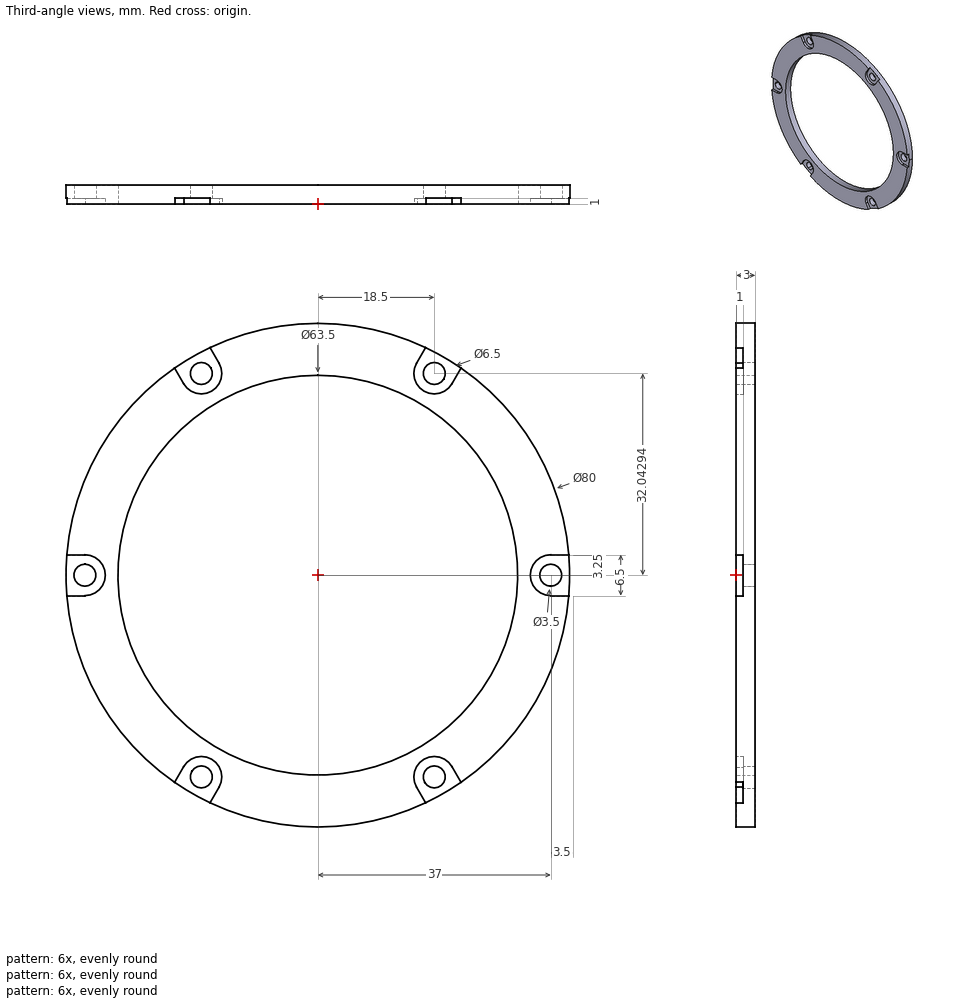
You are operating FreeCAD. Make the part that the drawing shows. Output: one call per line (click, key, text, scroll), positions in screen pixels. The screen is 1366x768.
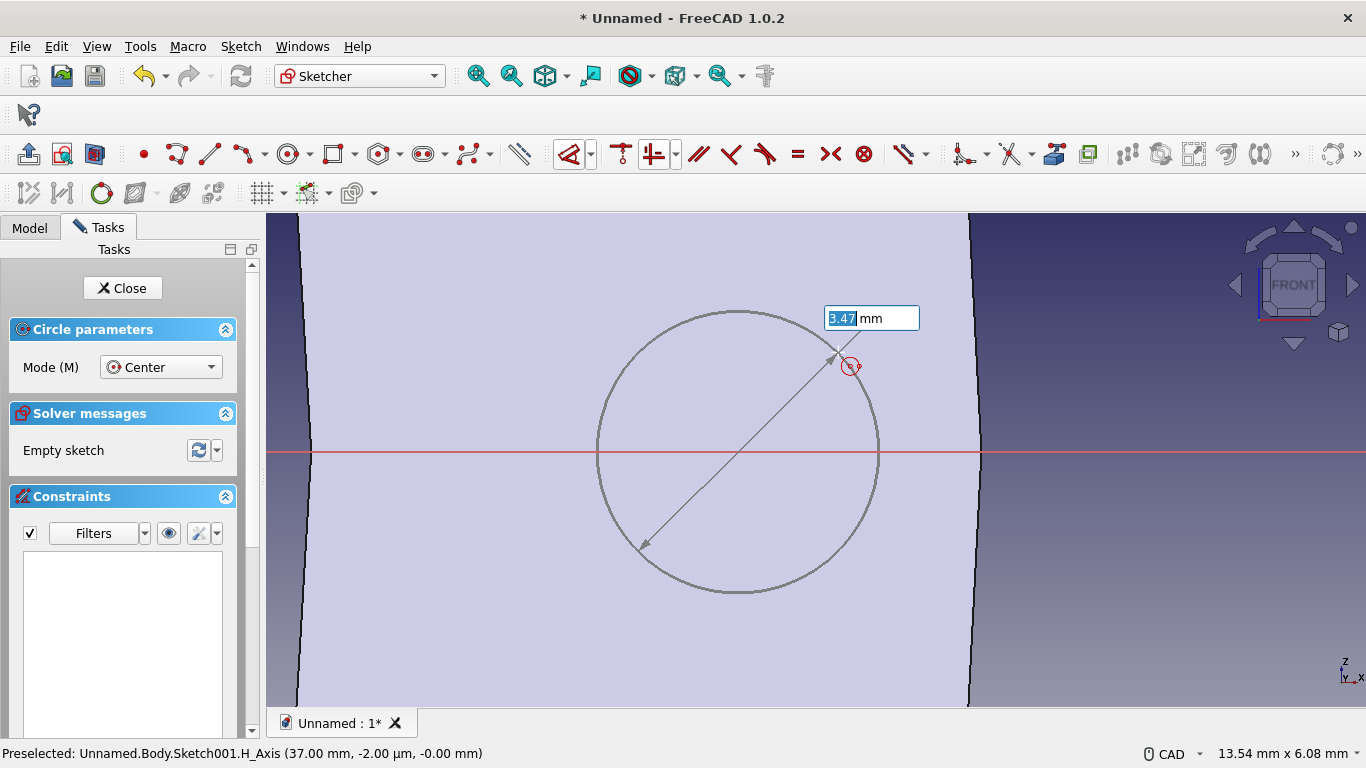
text(3.5)
key(Return)
key(Escape)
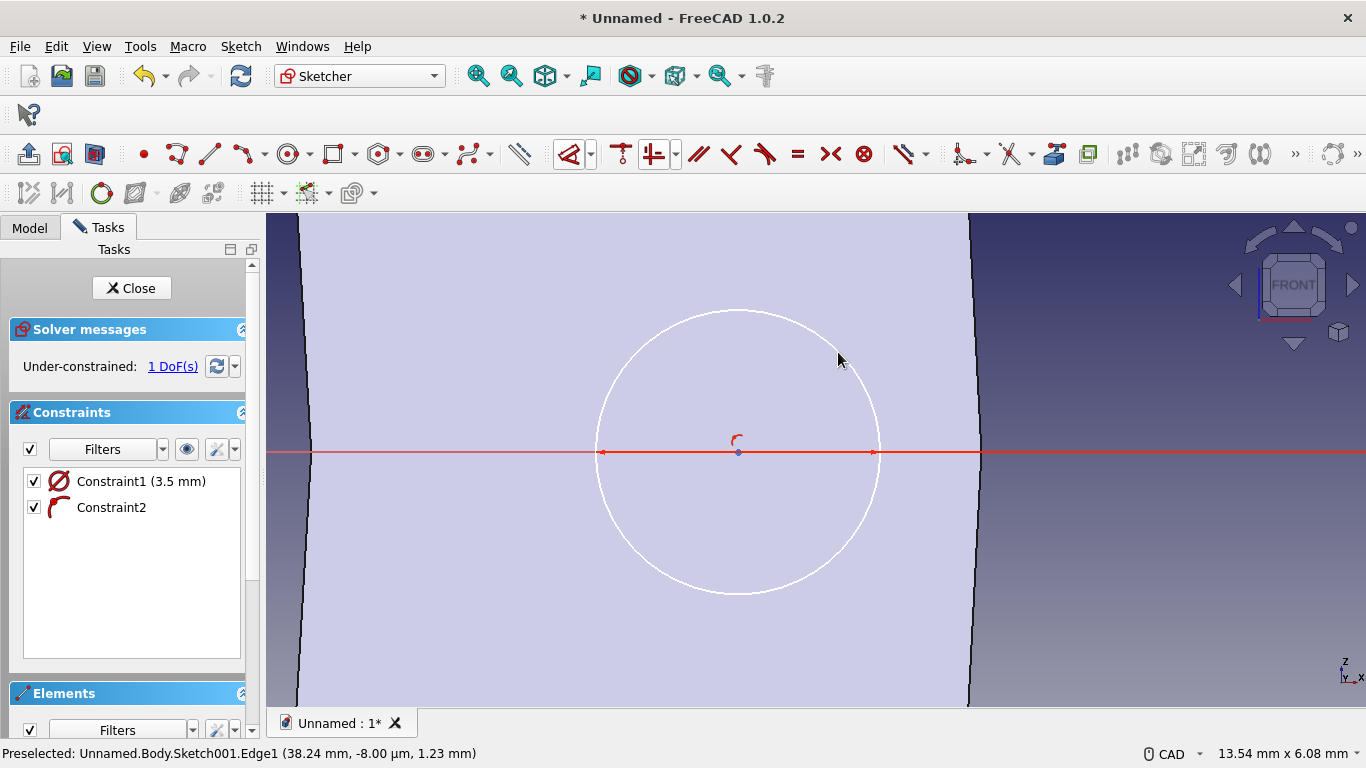
click(568, 154)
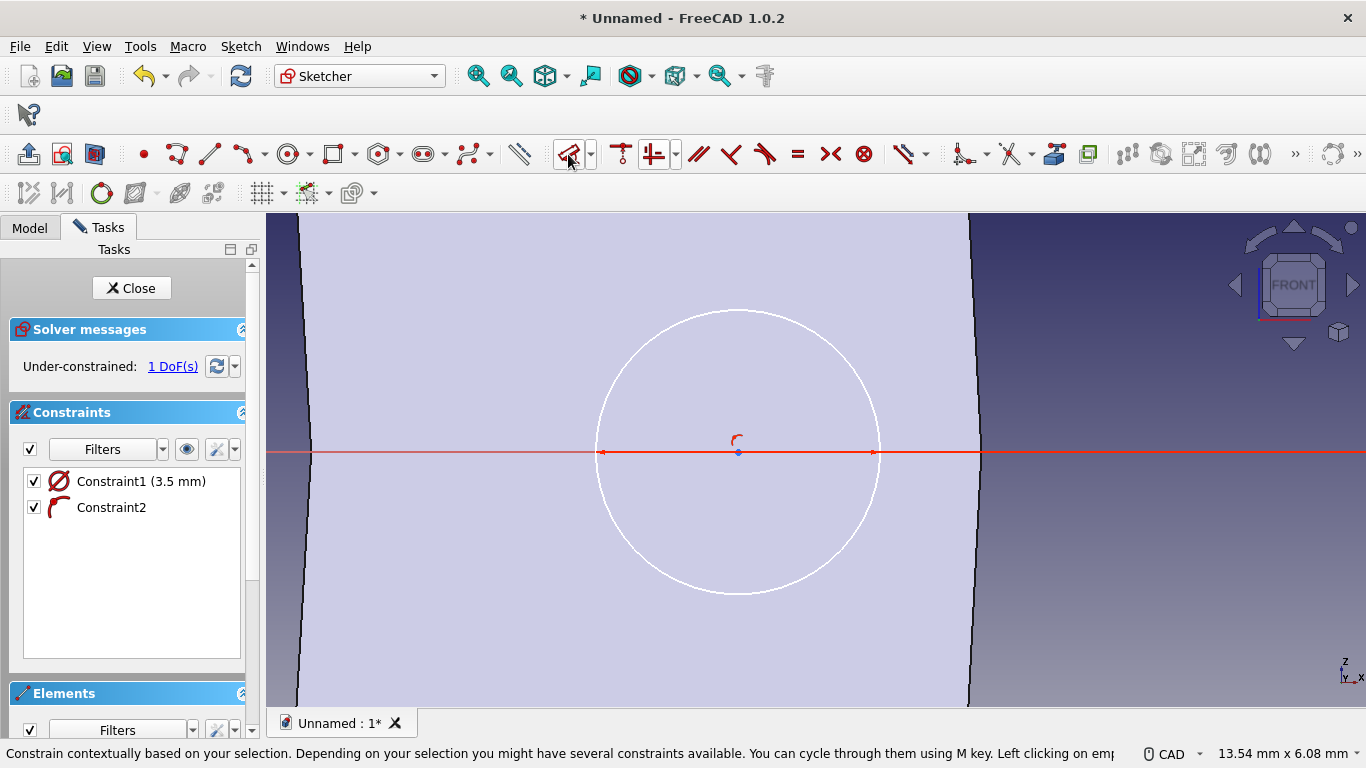
click(738, 452)
click(516, 486)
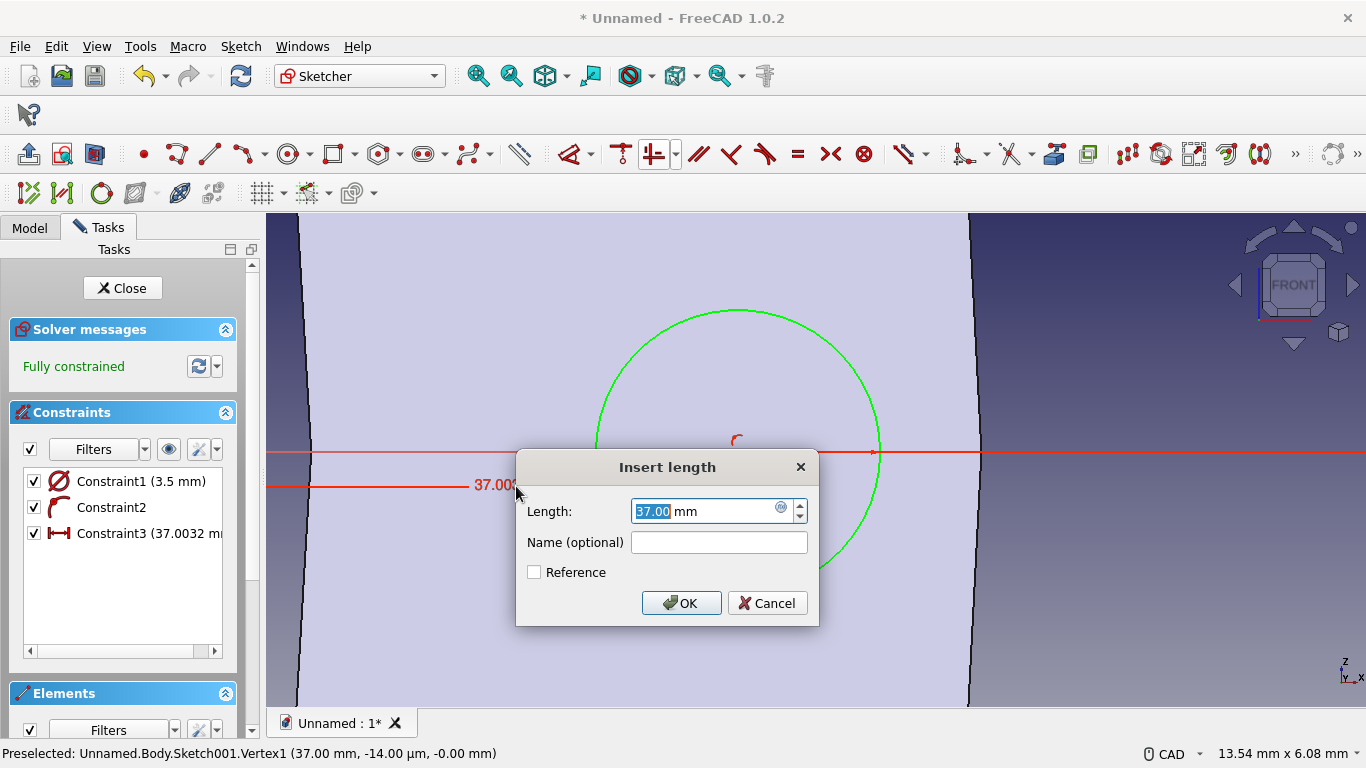
text(37)
key(Return)
key(Escape)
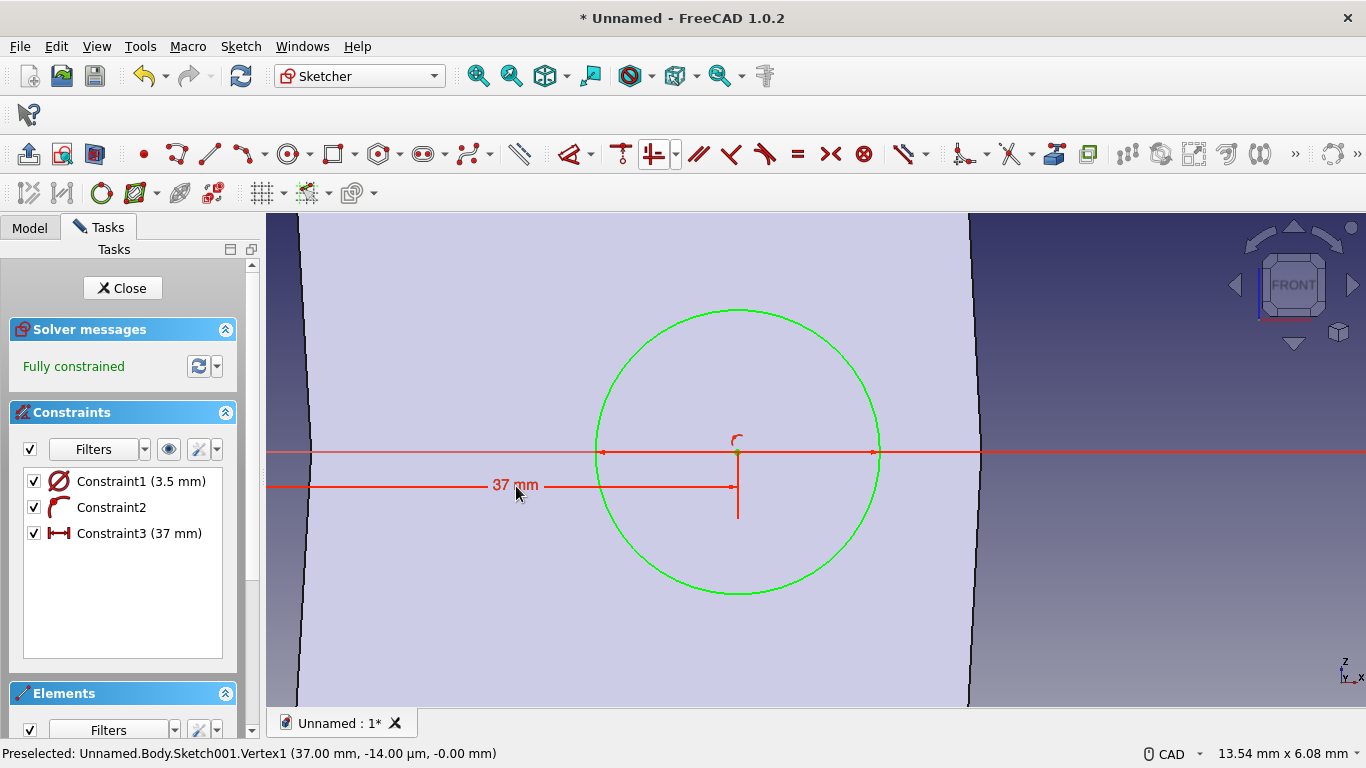
click(123, 288)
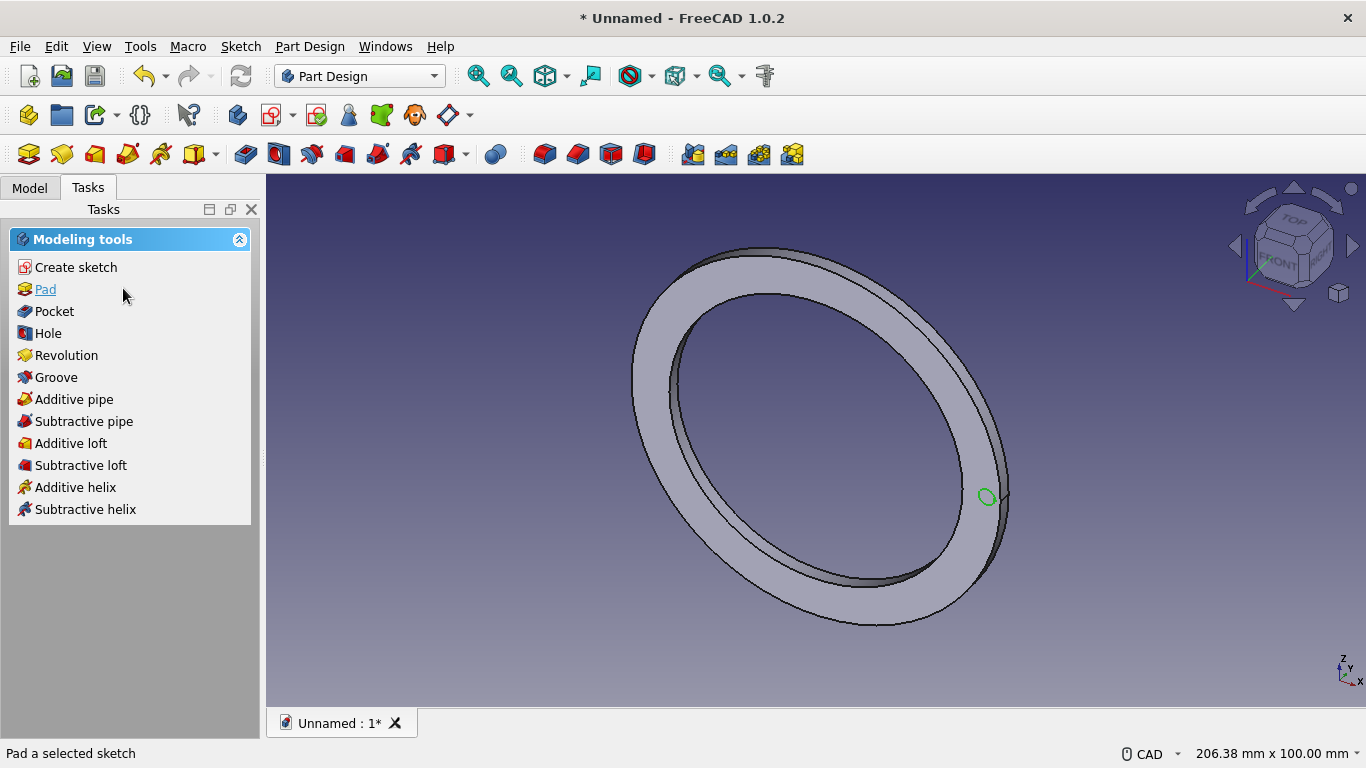
click(246, 154)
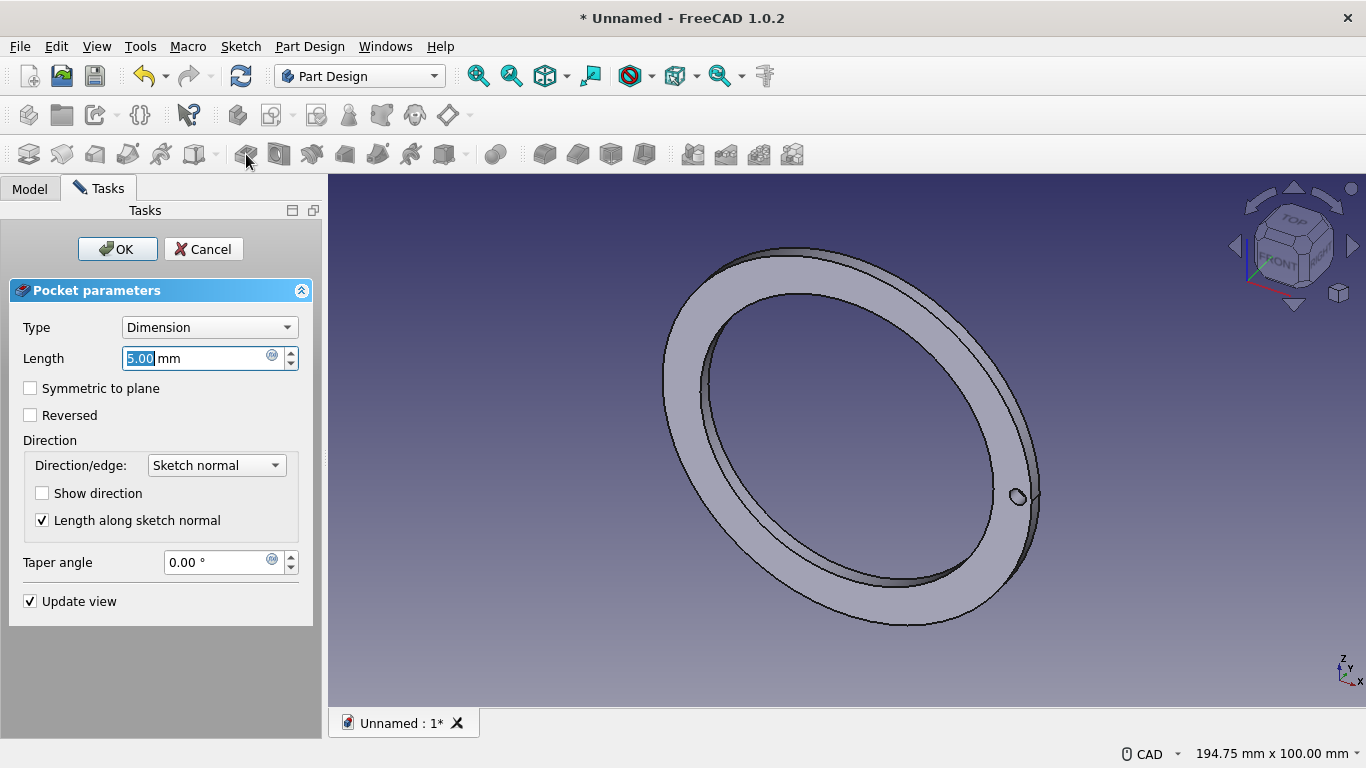
click(210, 328)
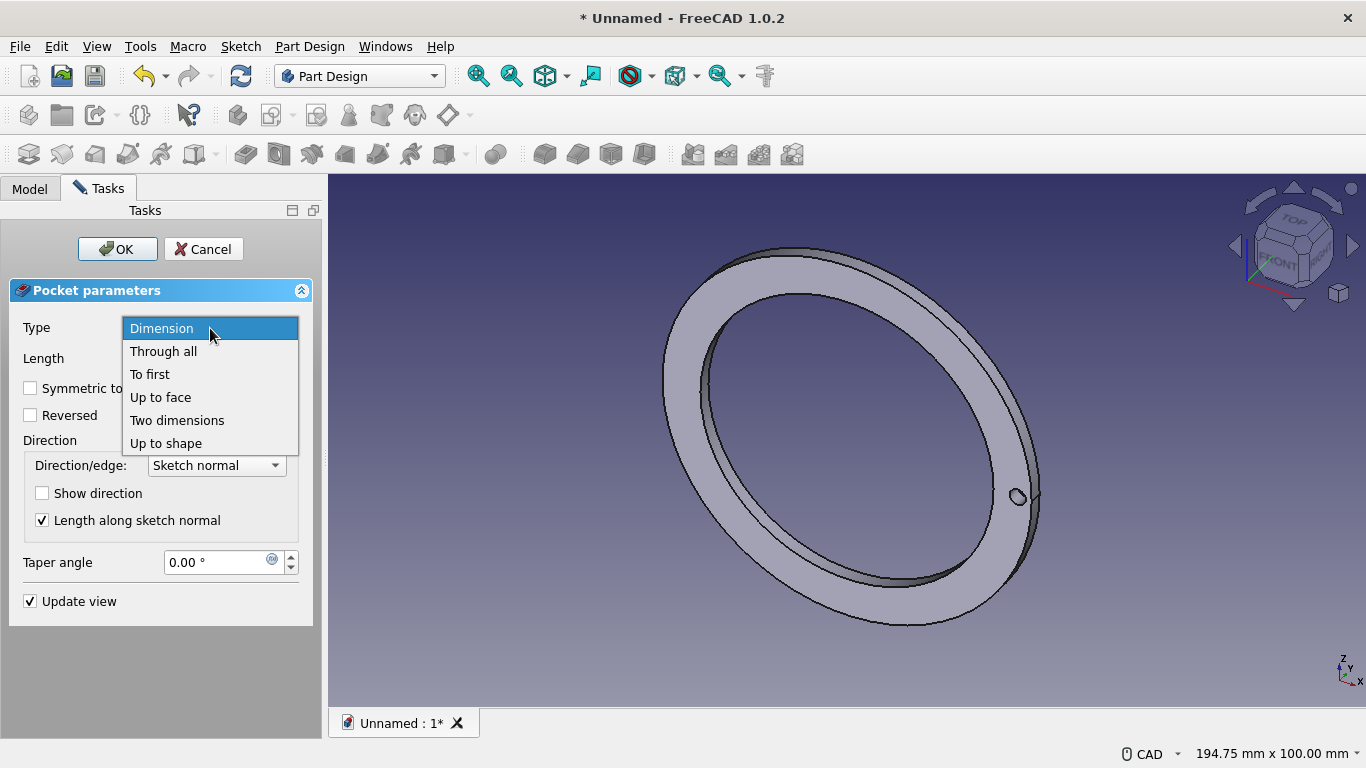
click(208, 352)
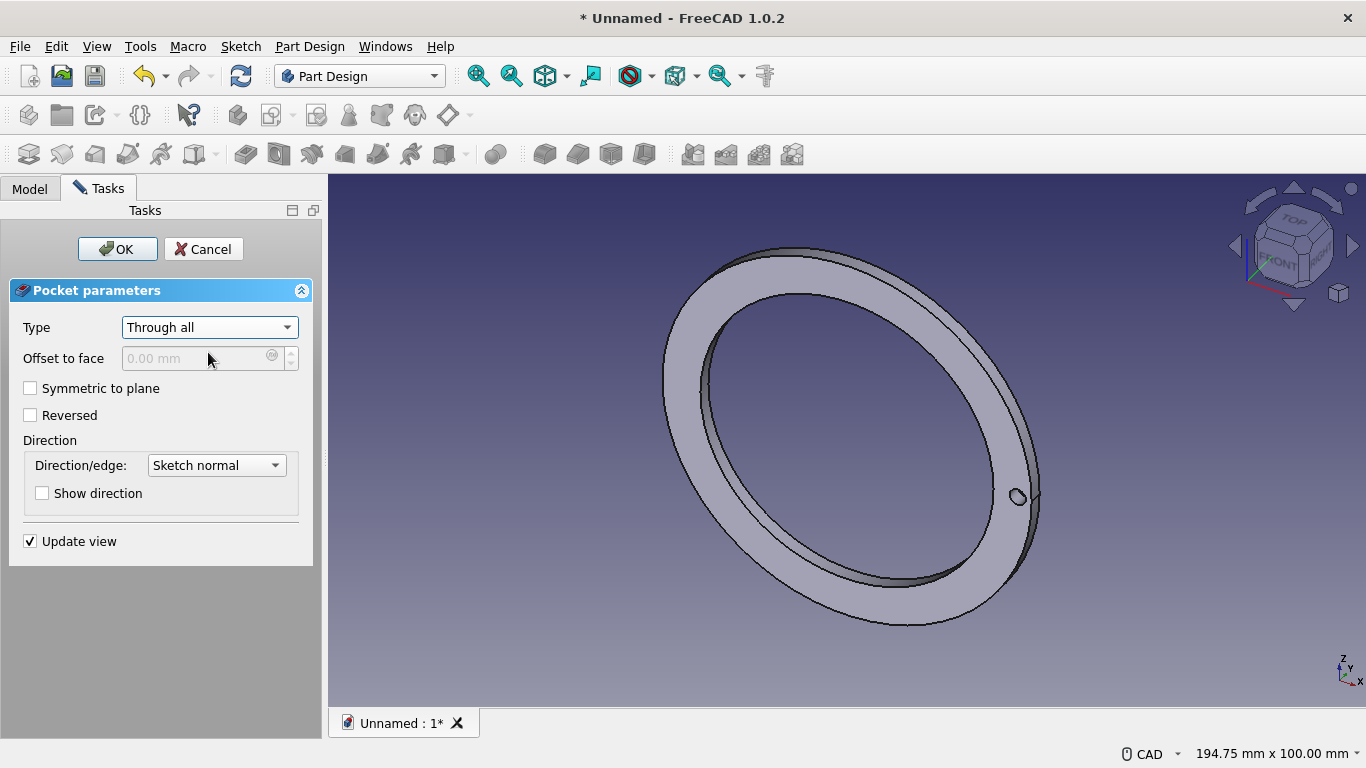
click(118, 249)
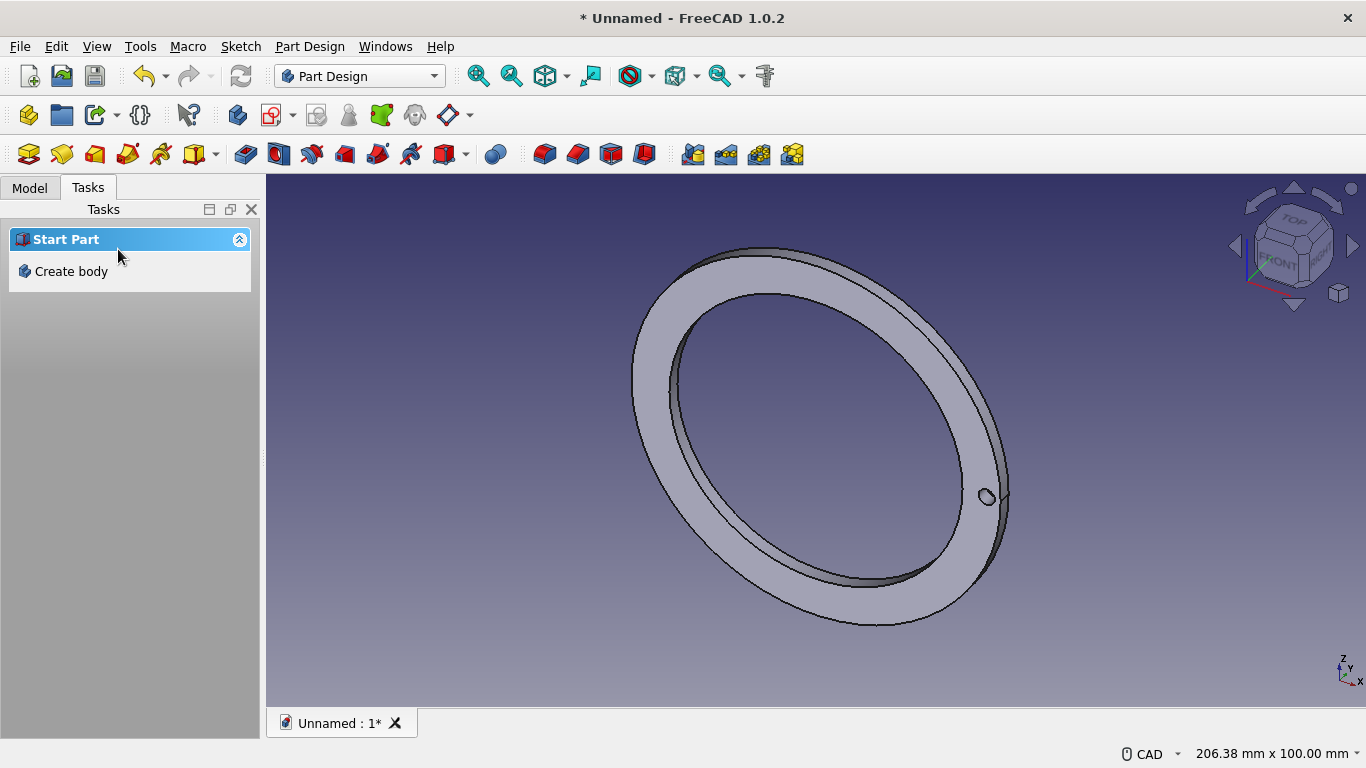
click(30, 188)